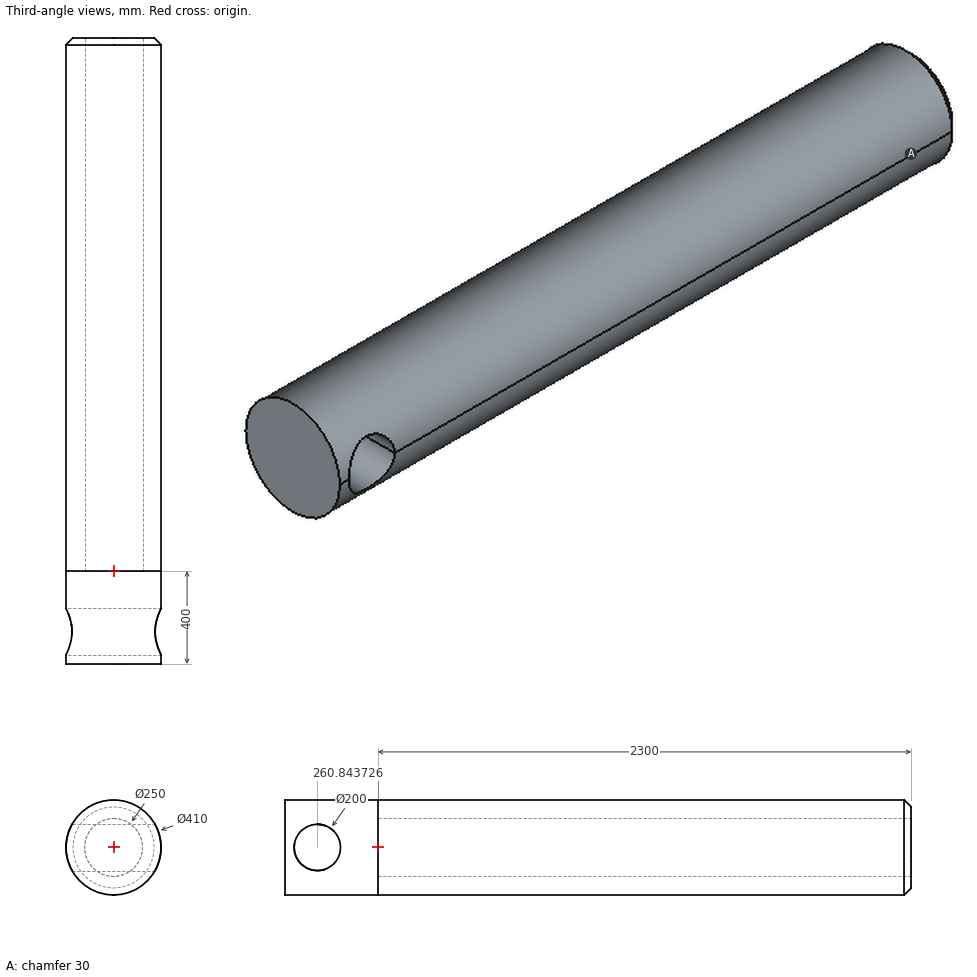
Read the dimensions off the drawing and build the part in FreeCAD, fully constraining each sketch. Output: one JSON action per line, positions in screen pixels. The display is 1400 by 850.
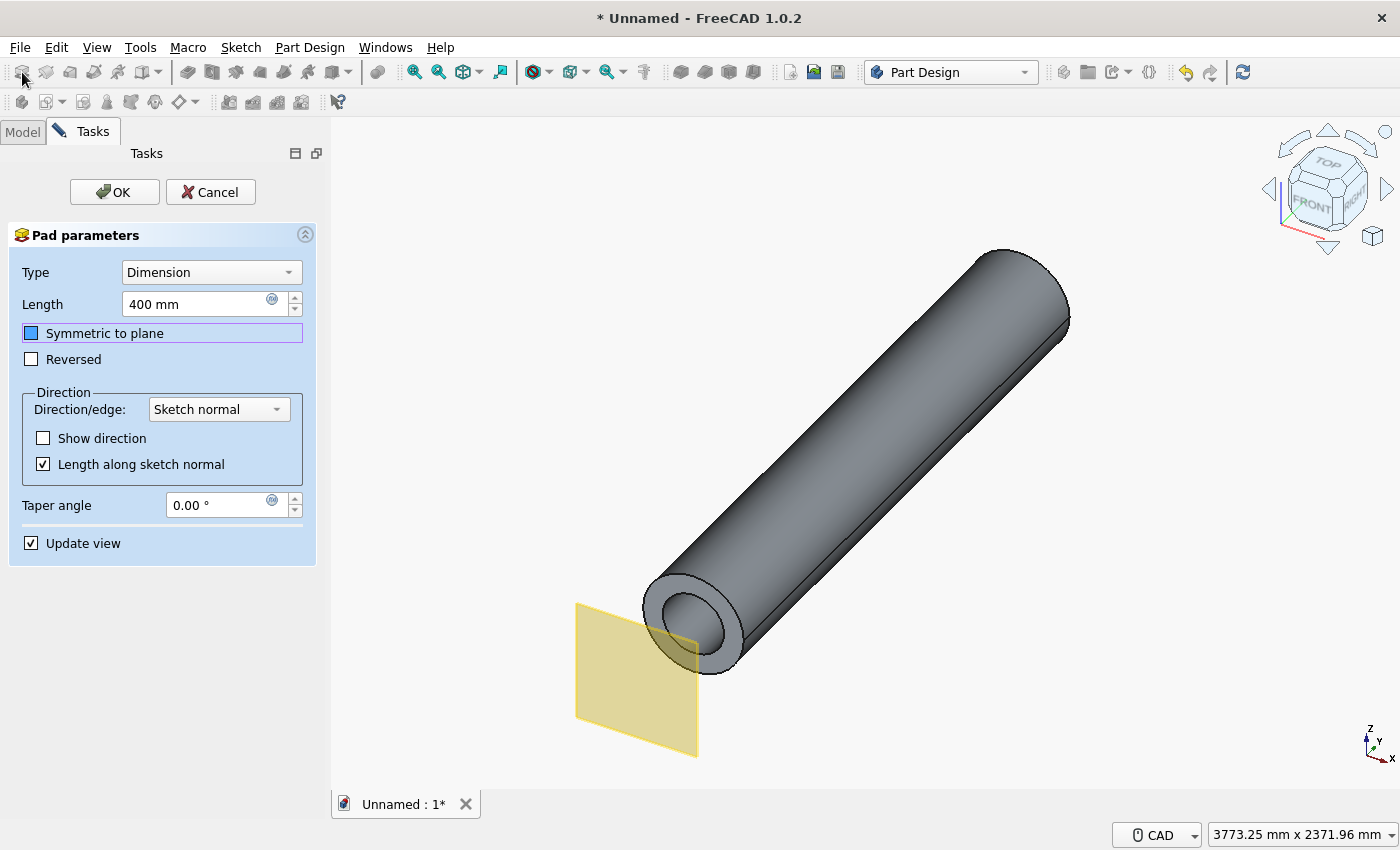
{"action": "left_click", "coordinate": [30, 359]}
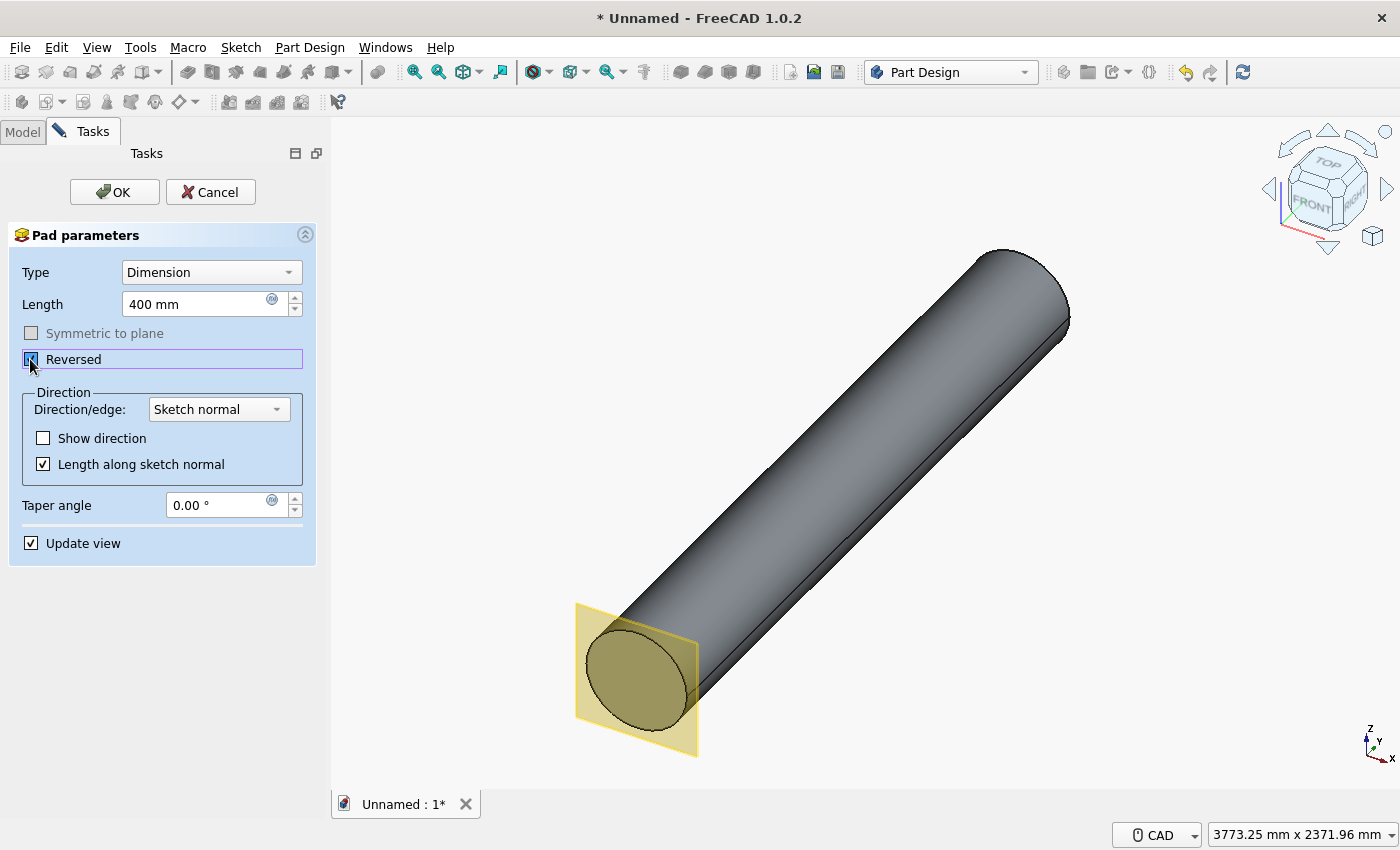
{"action": "left_click", "coordinate": [115, 192]}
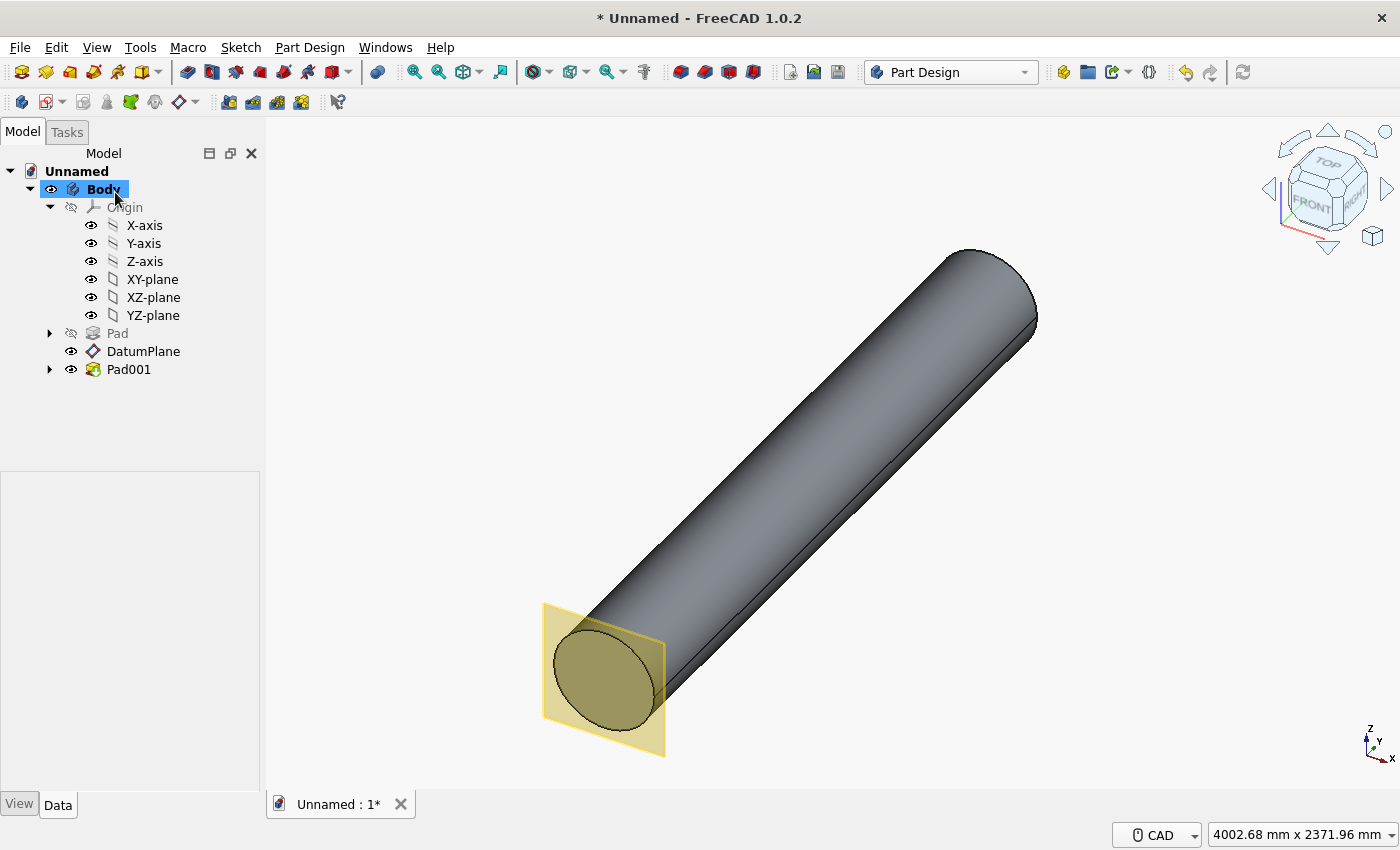
{"action": "left_click", "coordinate": [116, 351]}
{"action": "key", "text": "space"}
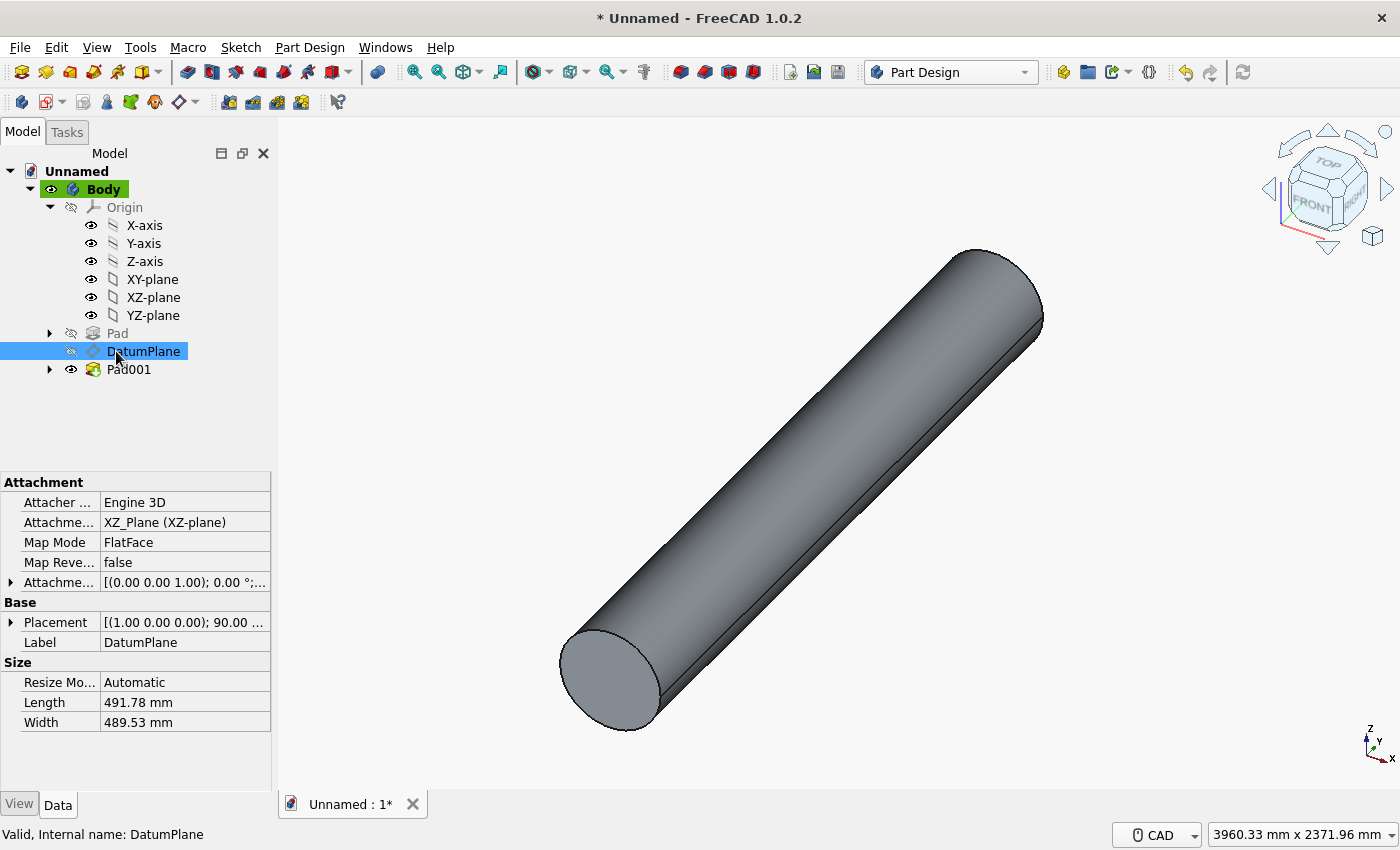
{"action": "left_click", "coordinate": [318, 749]}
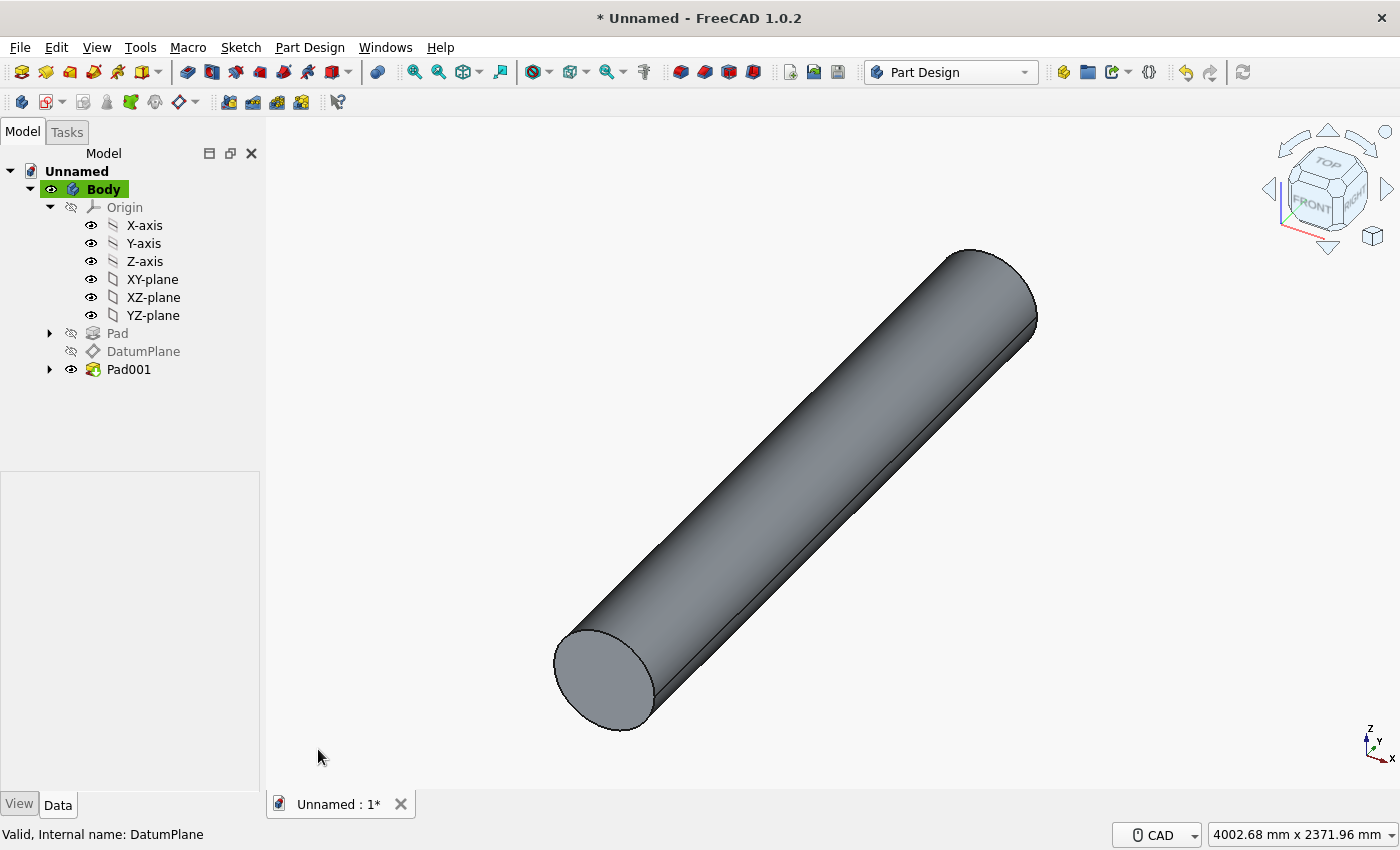
{"action": "left_click", "coordinate": [46, 102]}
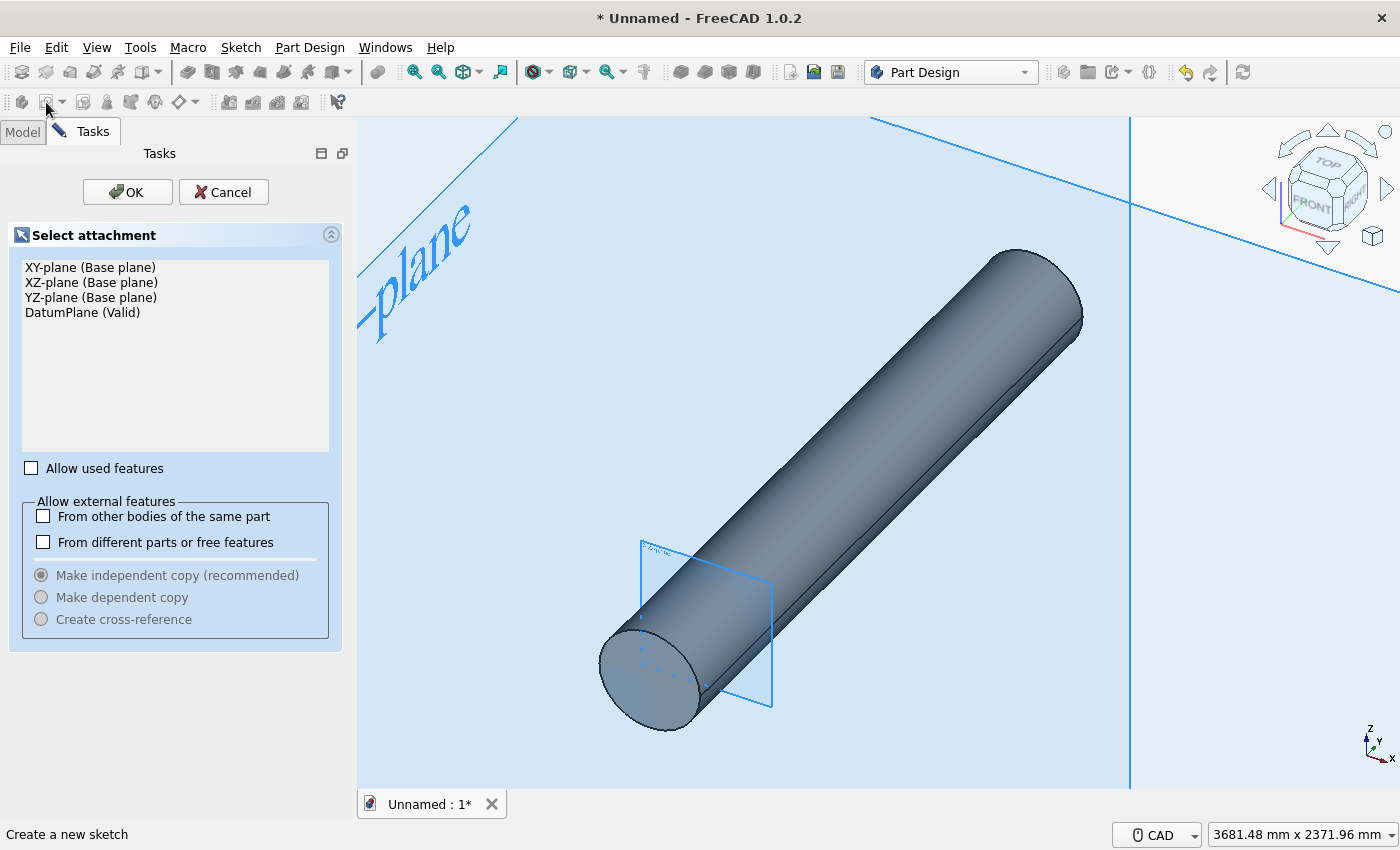
{"action": "left_click", "coordinate": [82, 298]}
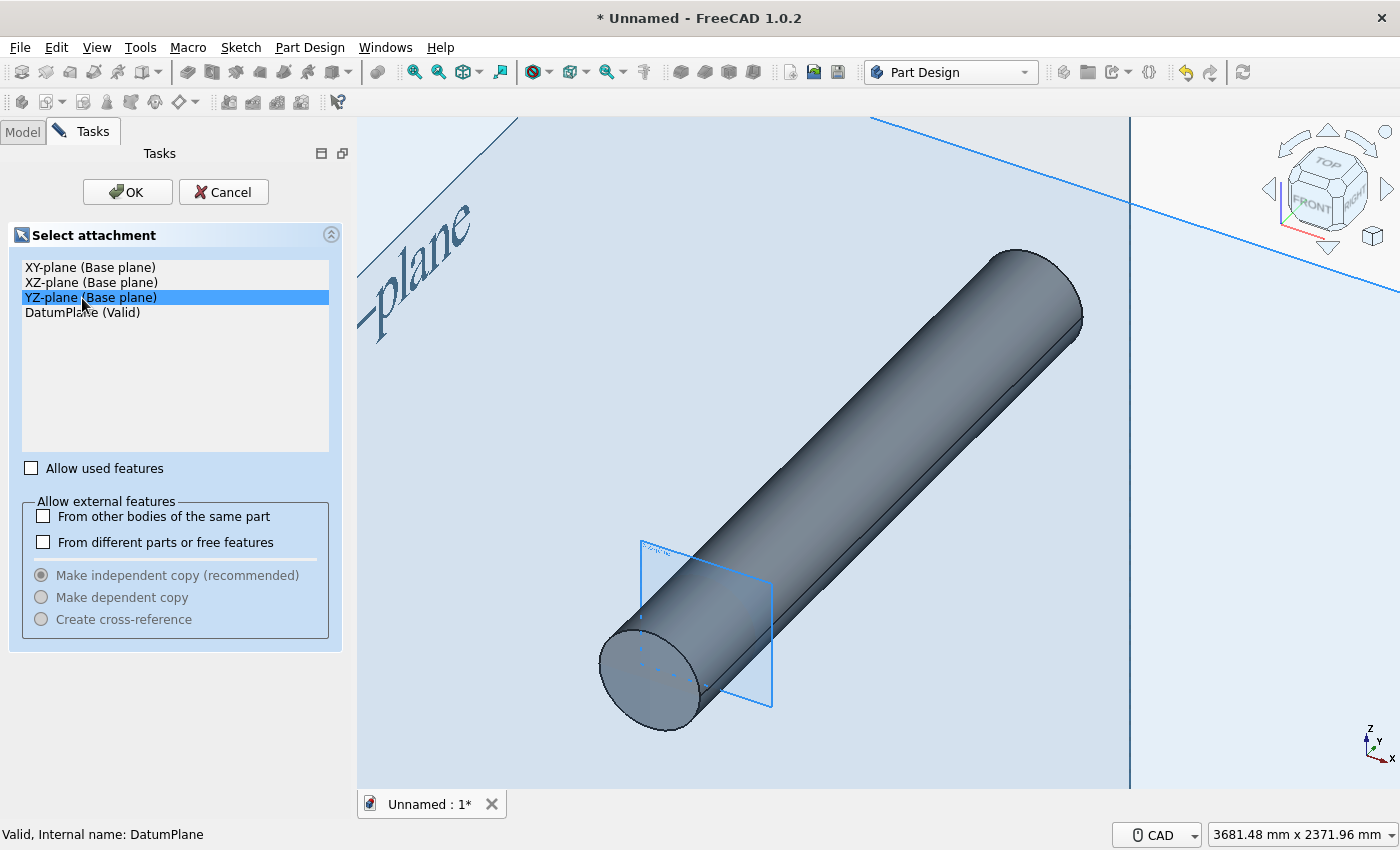
{"action": "left_click", "coordinate": [128, 192]}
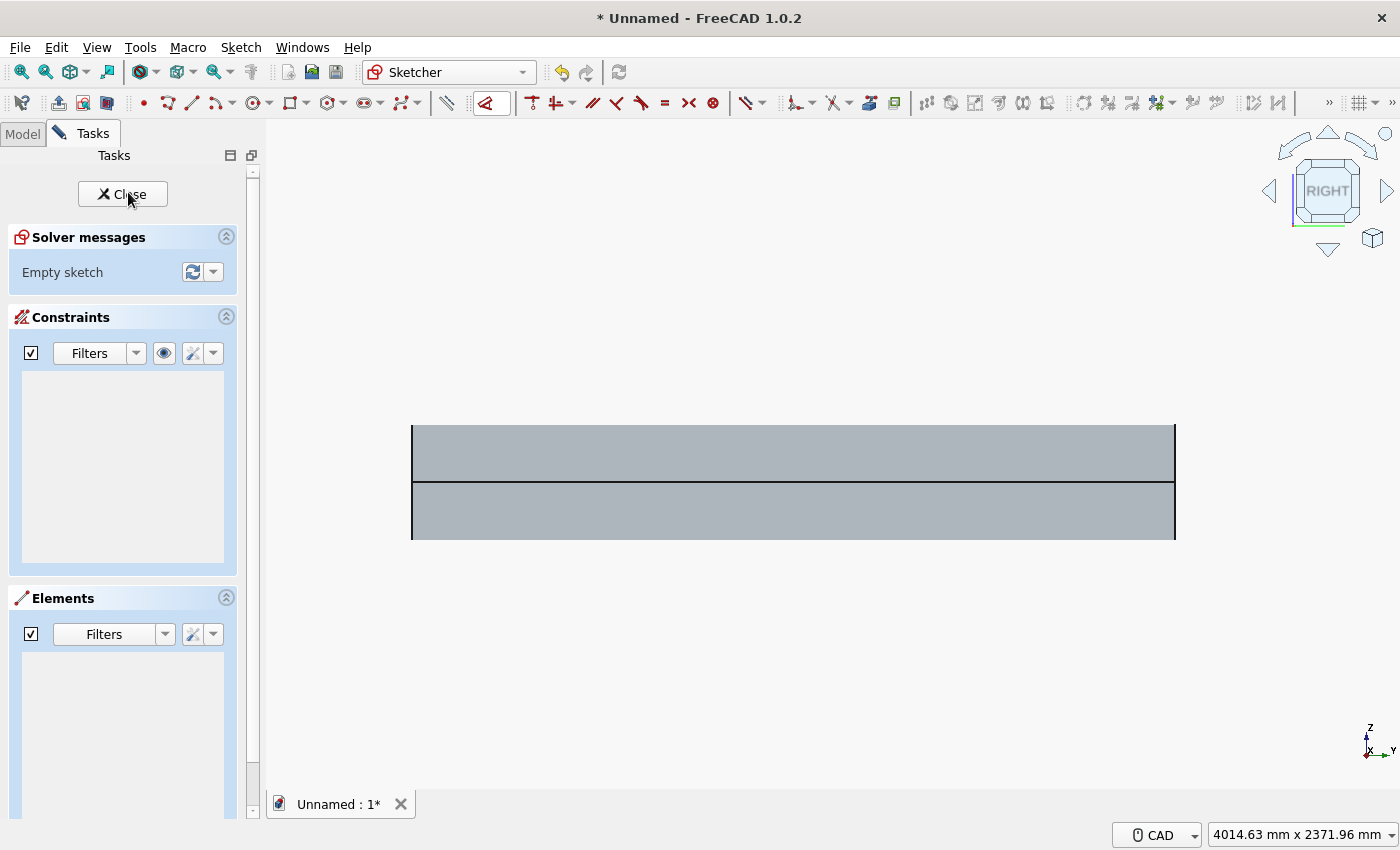
{"action": "left_click", "coordinate": [108, 104]}